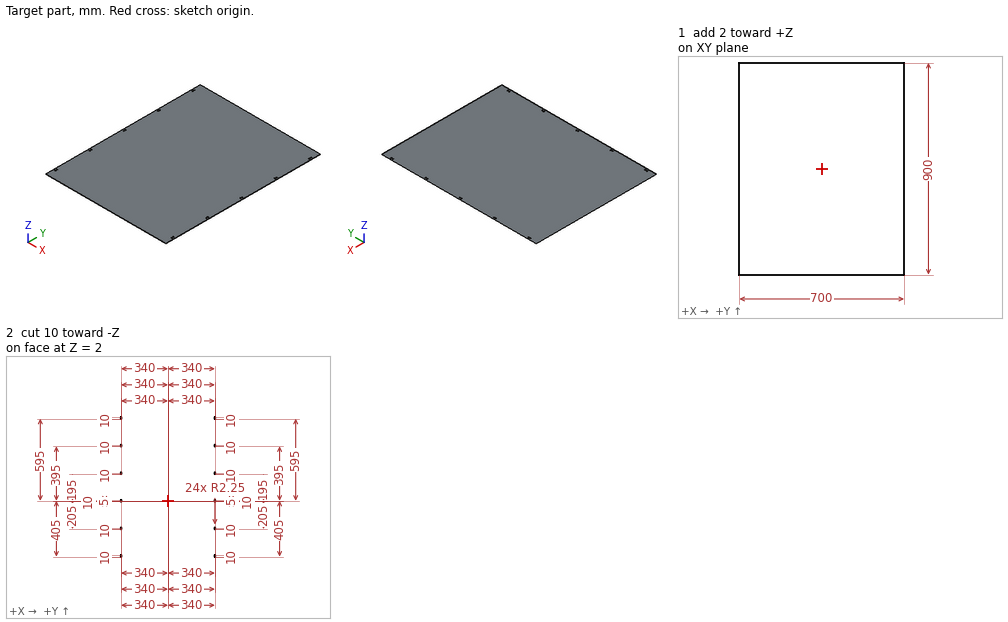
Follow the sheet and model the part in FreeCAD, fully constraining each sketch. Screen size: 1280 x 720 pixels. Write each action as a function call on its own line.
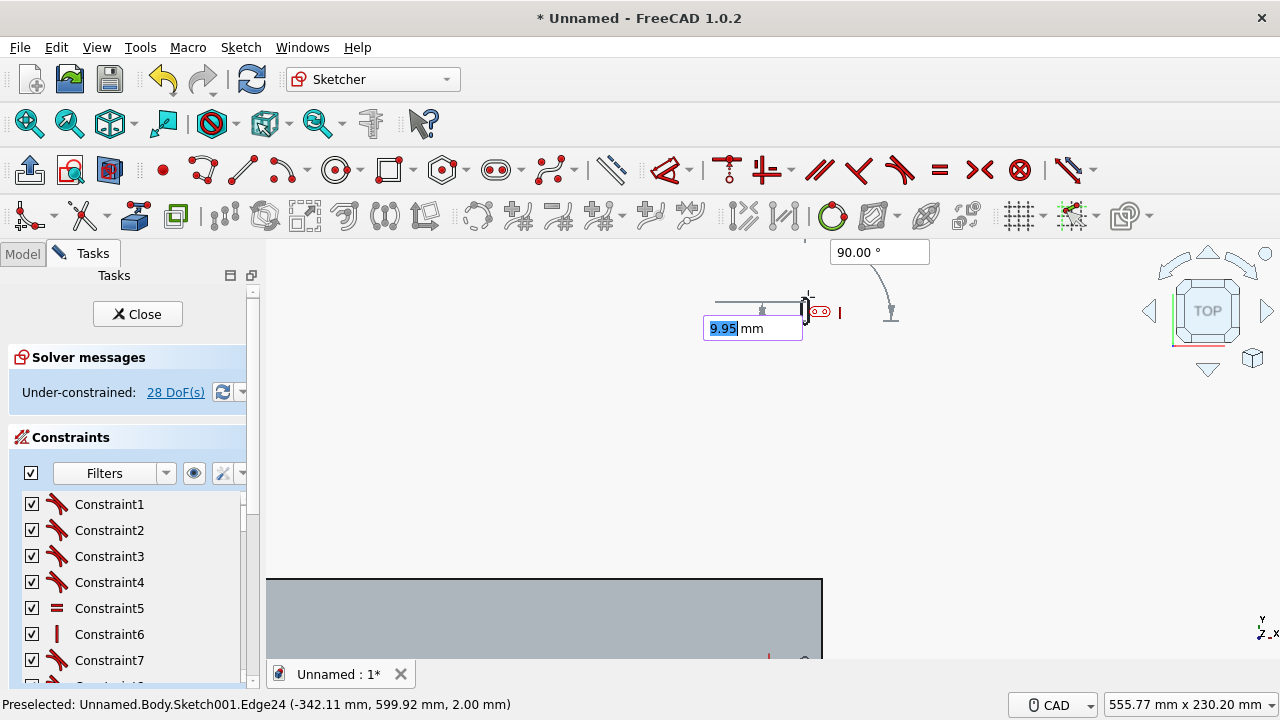
click(805, 296)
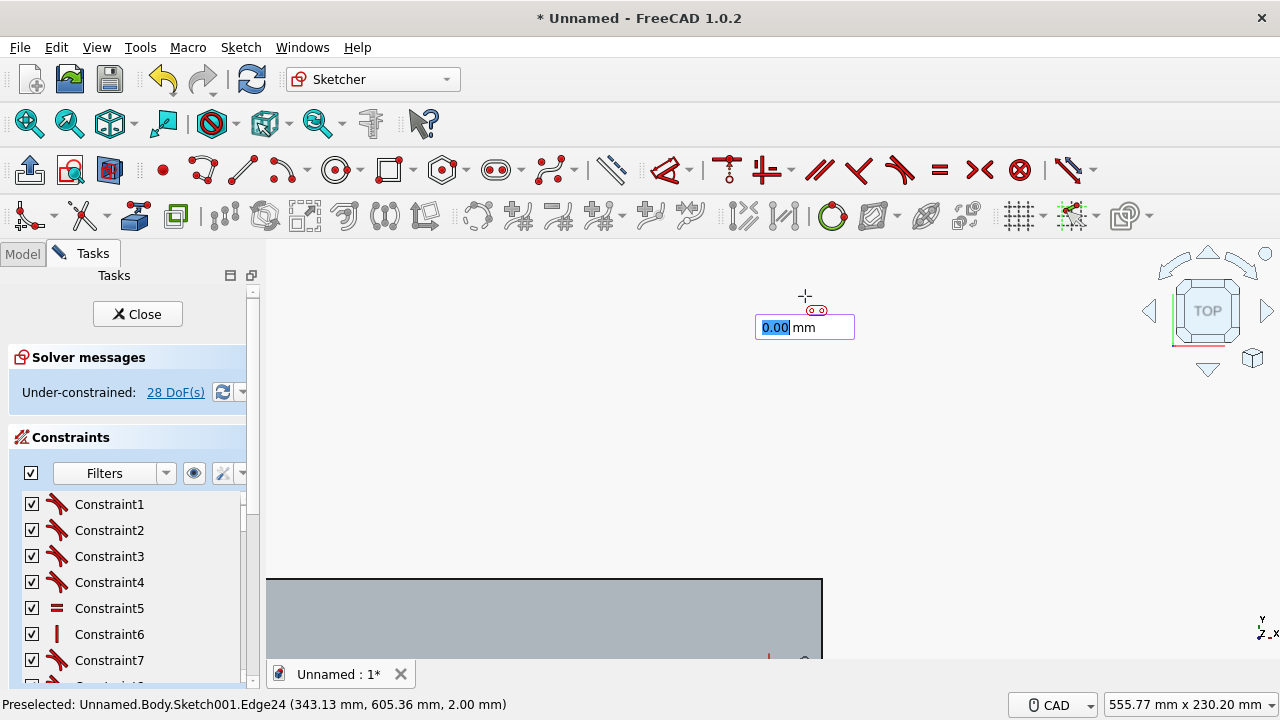
scroll(808, 305, up, 7)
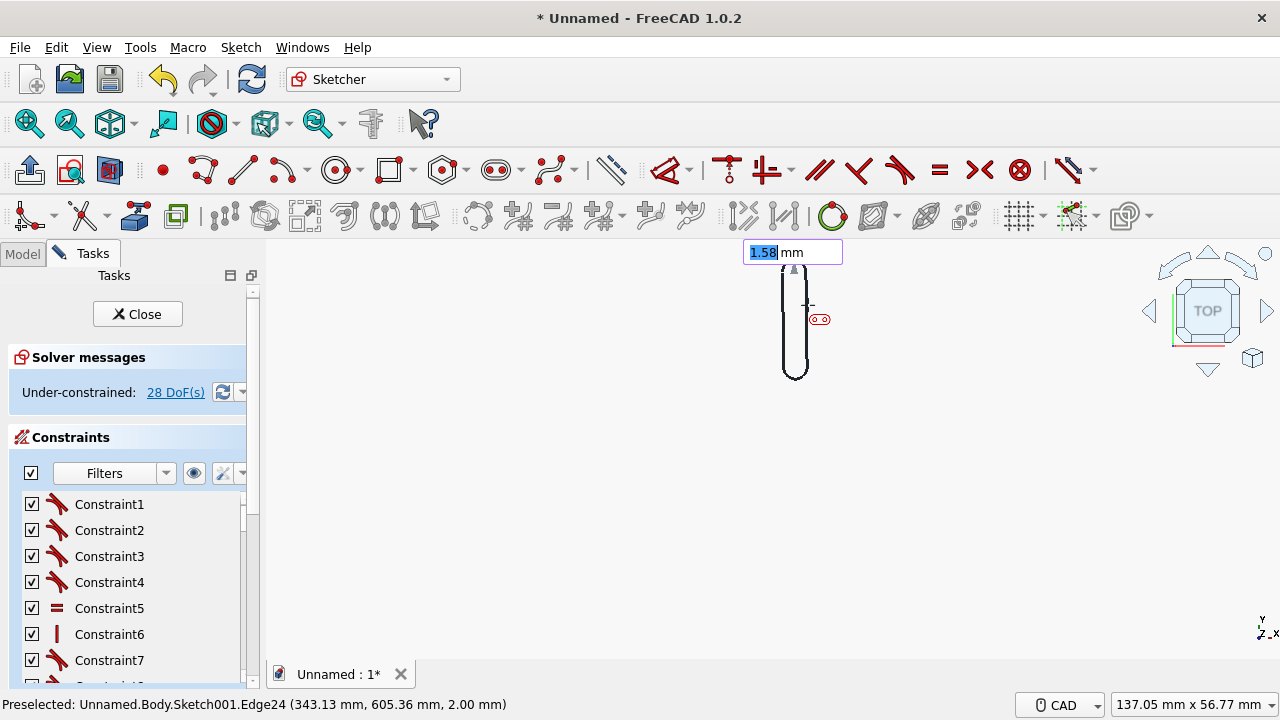
click(807, 306)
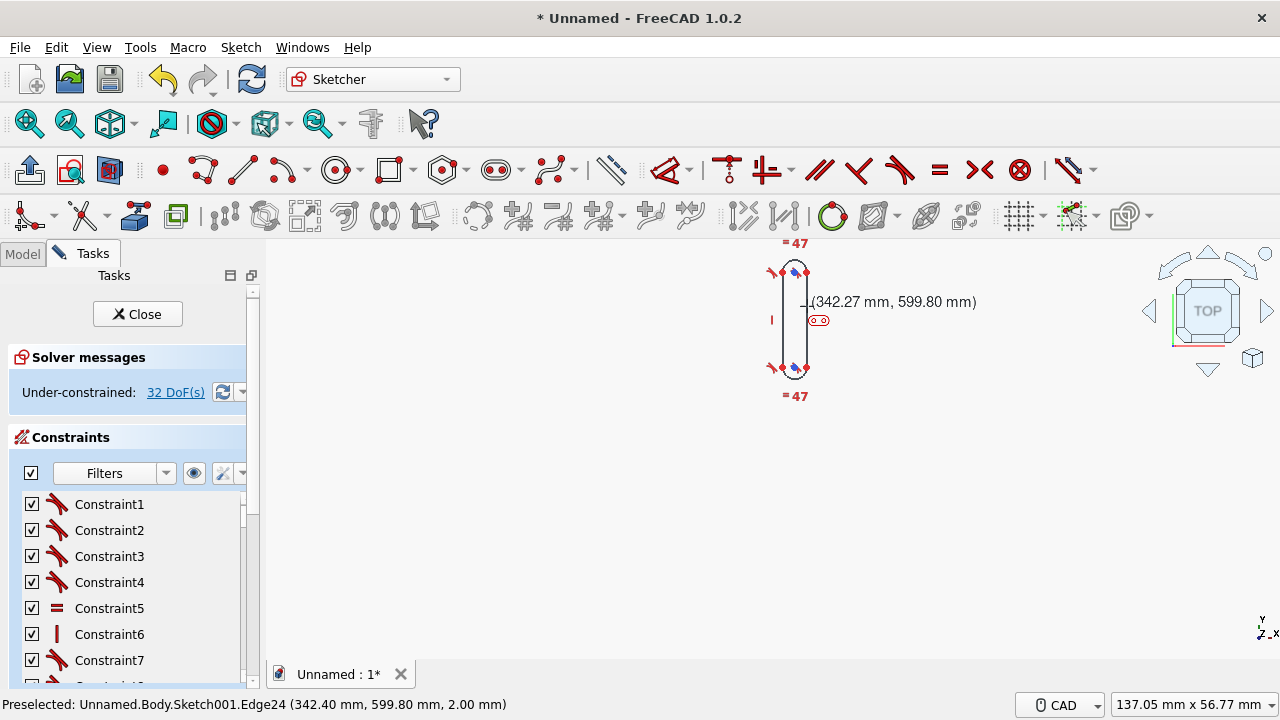
scroll(808, 298, down, 16)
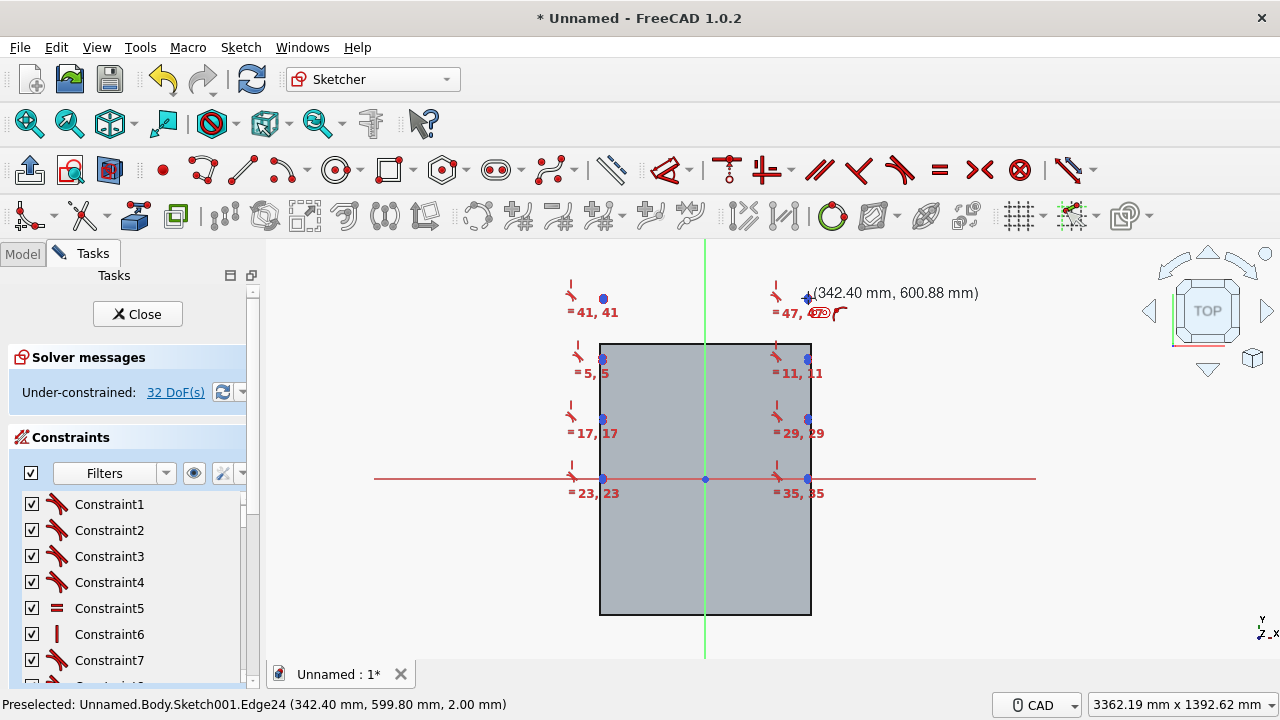
scroll(808, 541, up, 18)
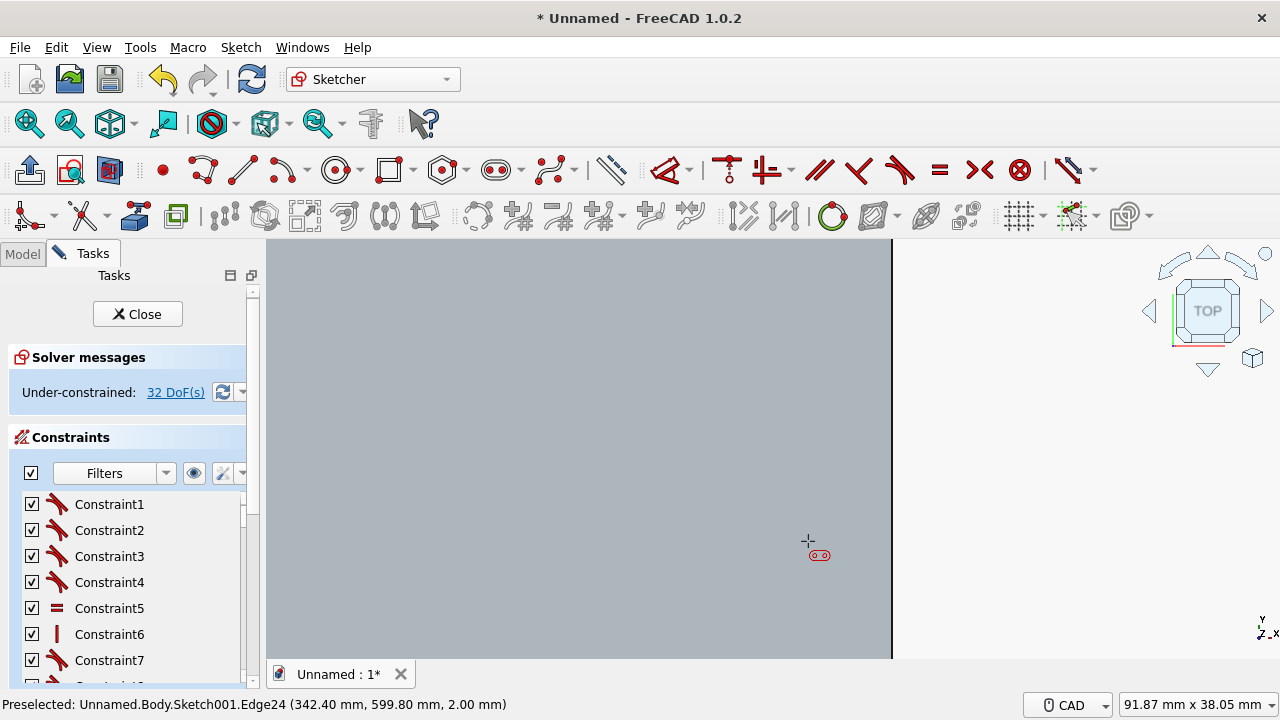
scroll(808, 541, down, 18)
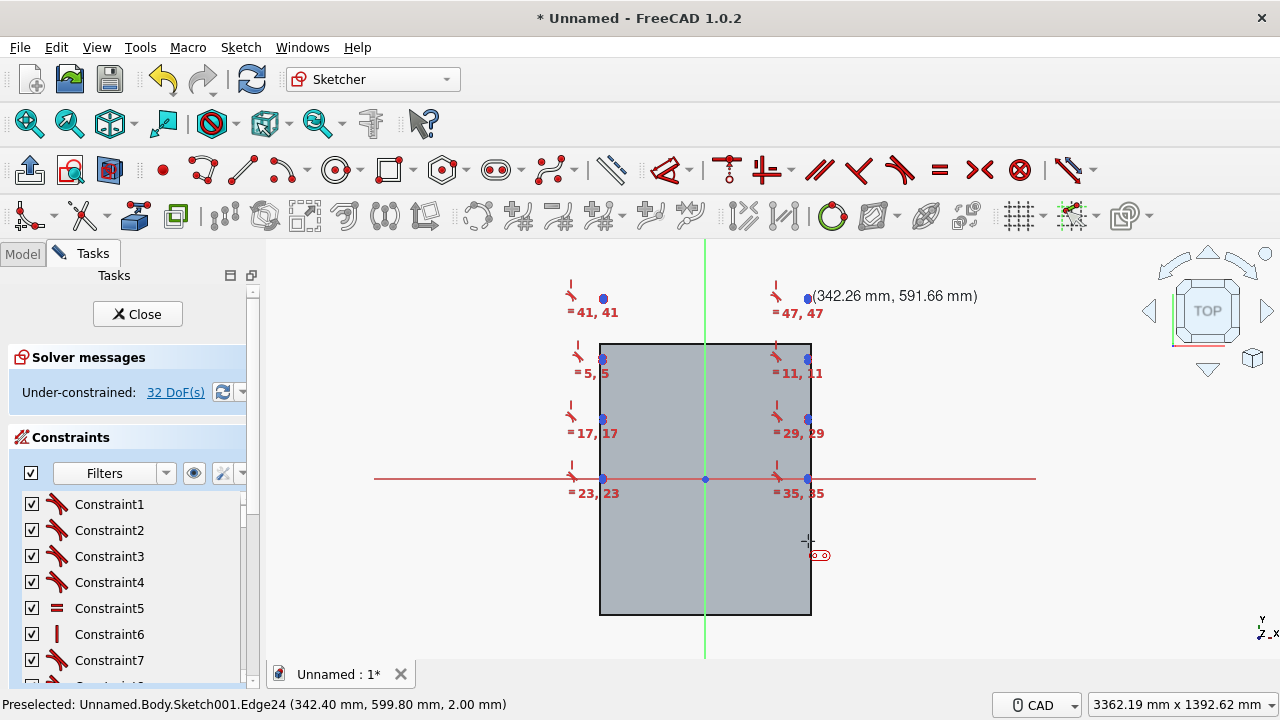
click(808, 541)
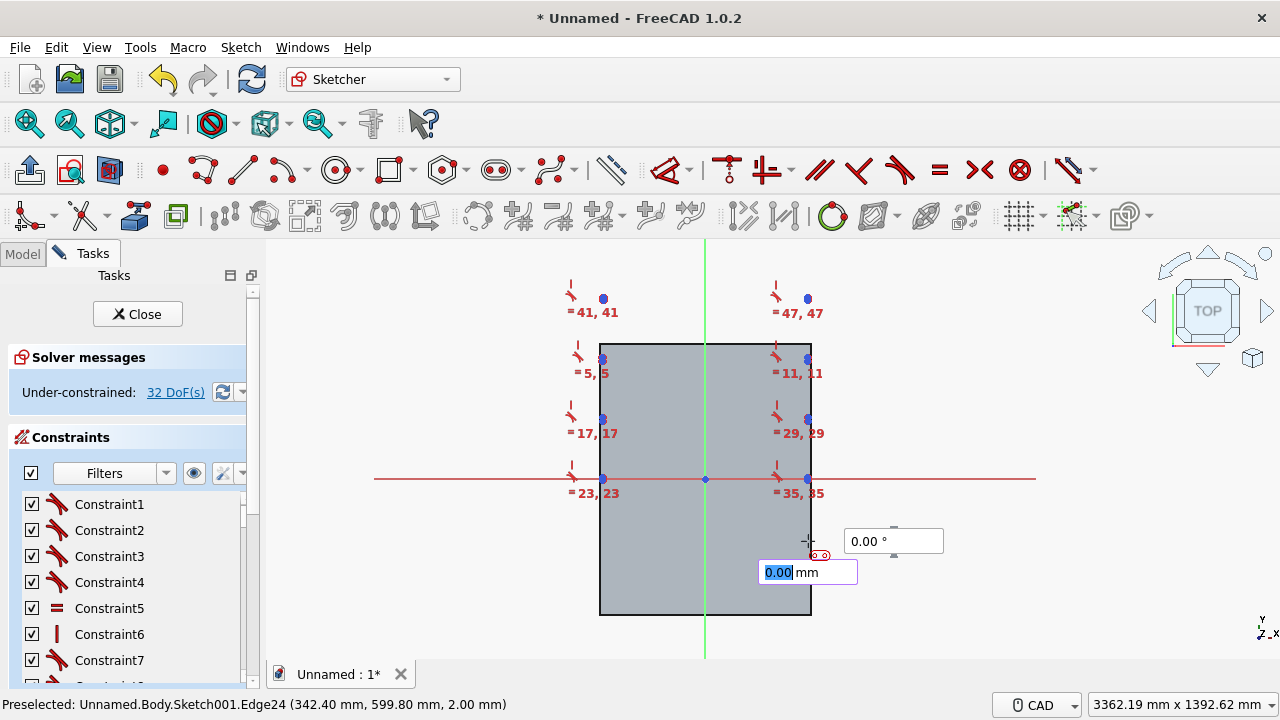
scroll(808, 538, up, 9)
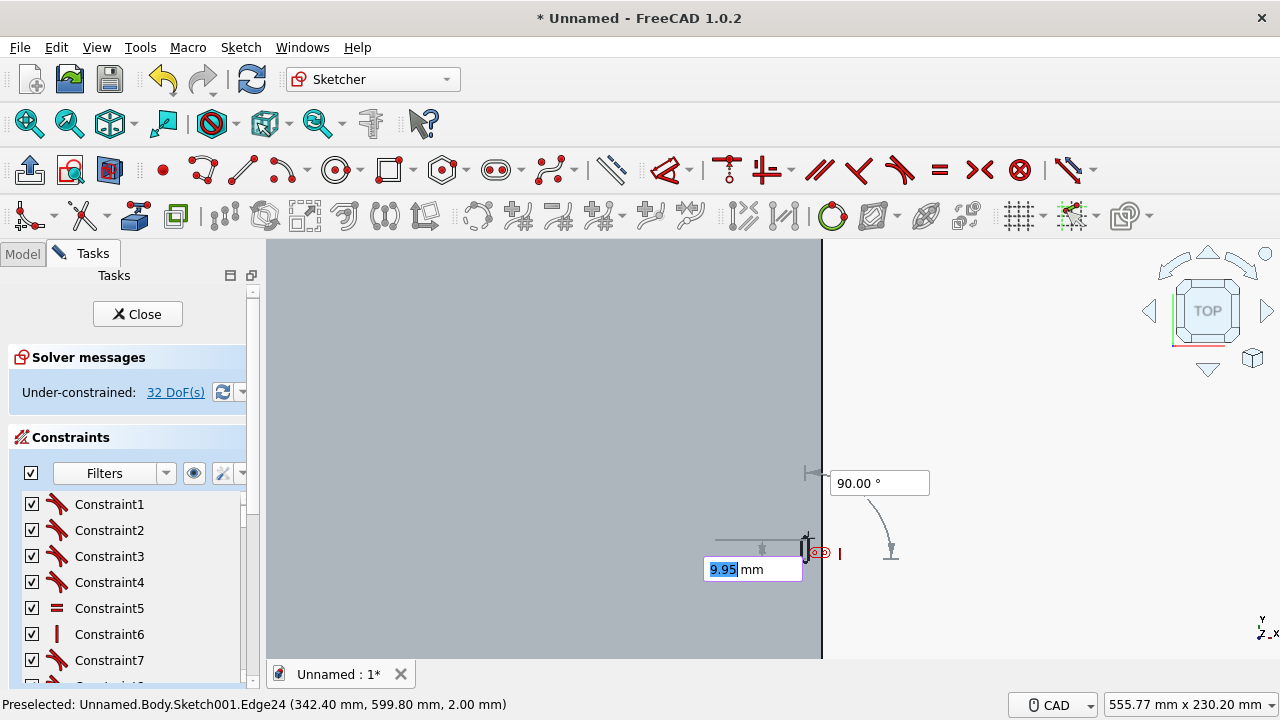
click(805, 536)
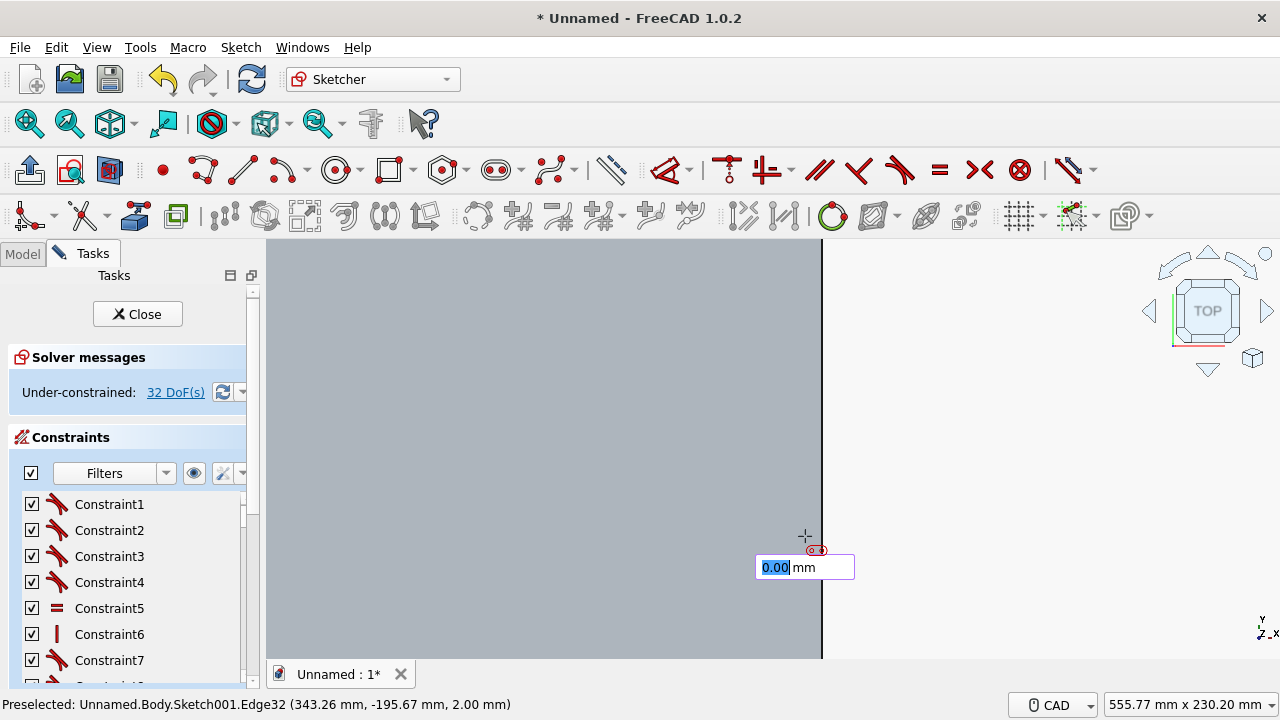
scroll(808, 545, up, 7)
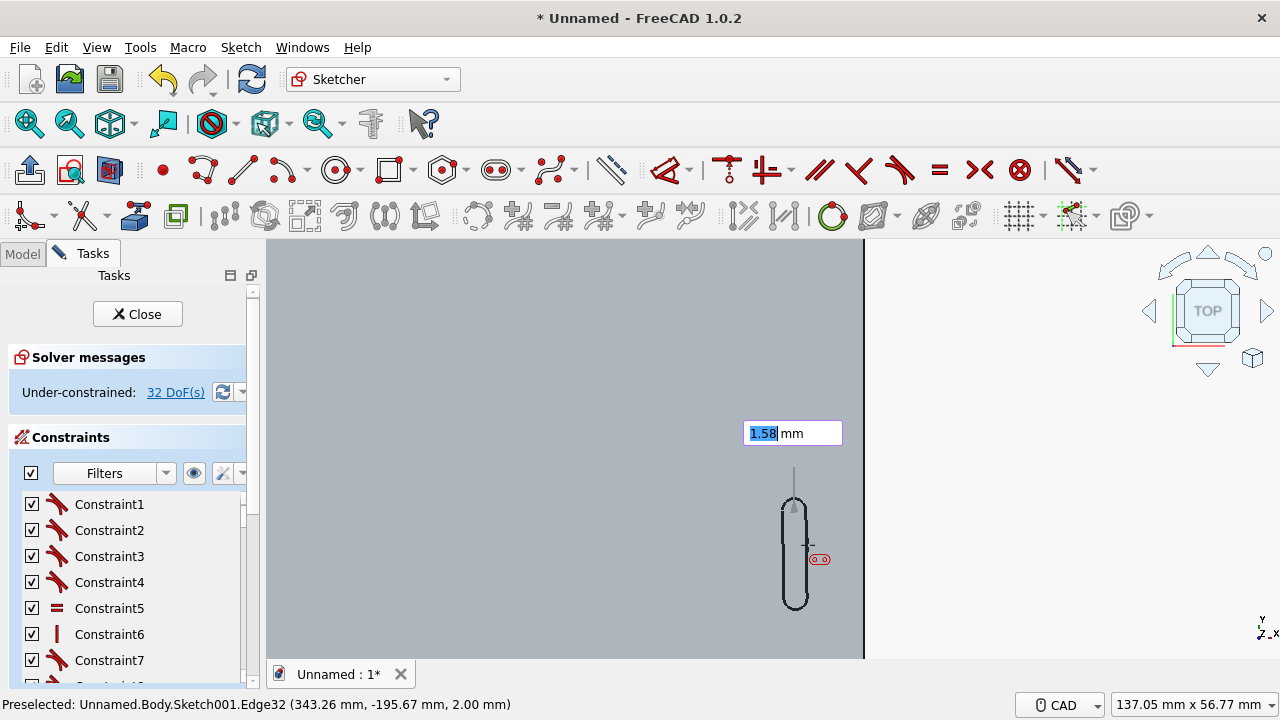
click(807, 542)